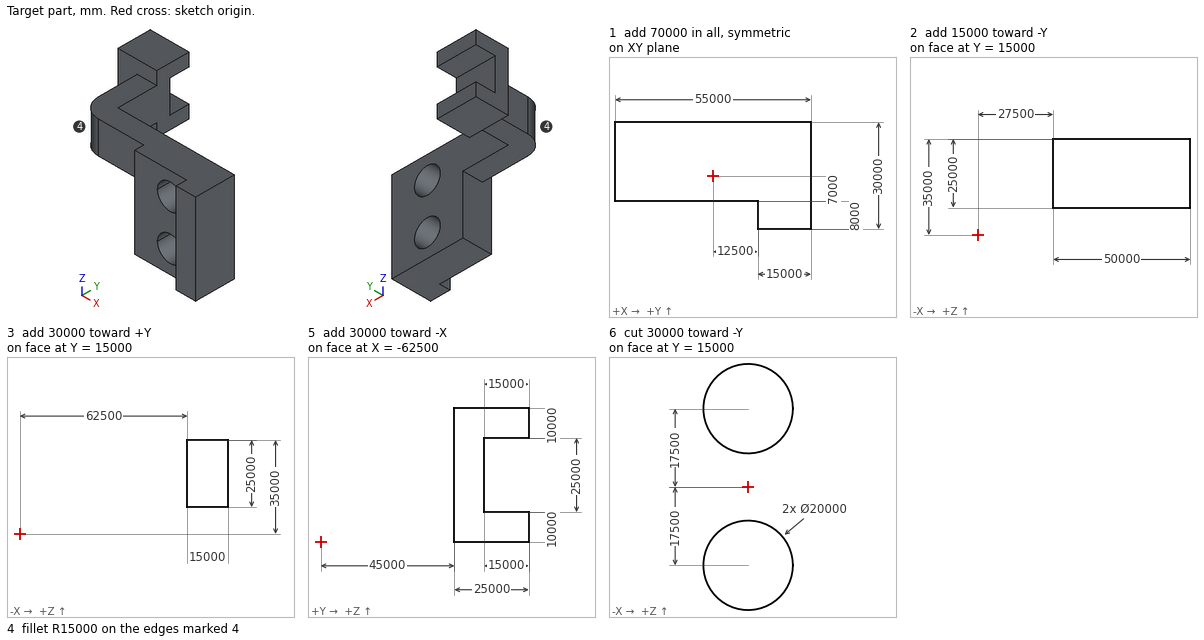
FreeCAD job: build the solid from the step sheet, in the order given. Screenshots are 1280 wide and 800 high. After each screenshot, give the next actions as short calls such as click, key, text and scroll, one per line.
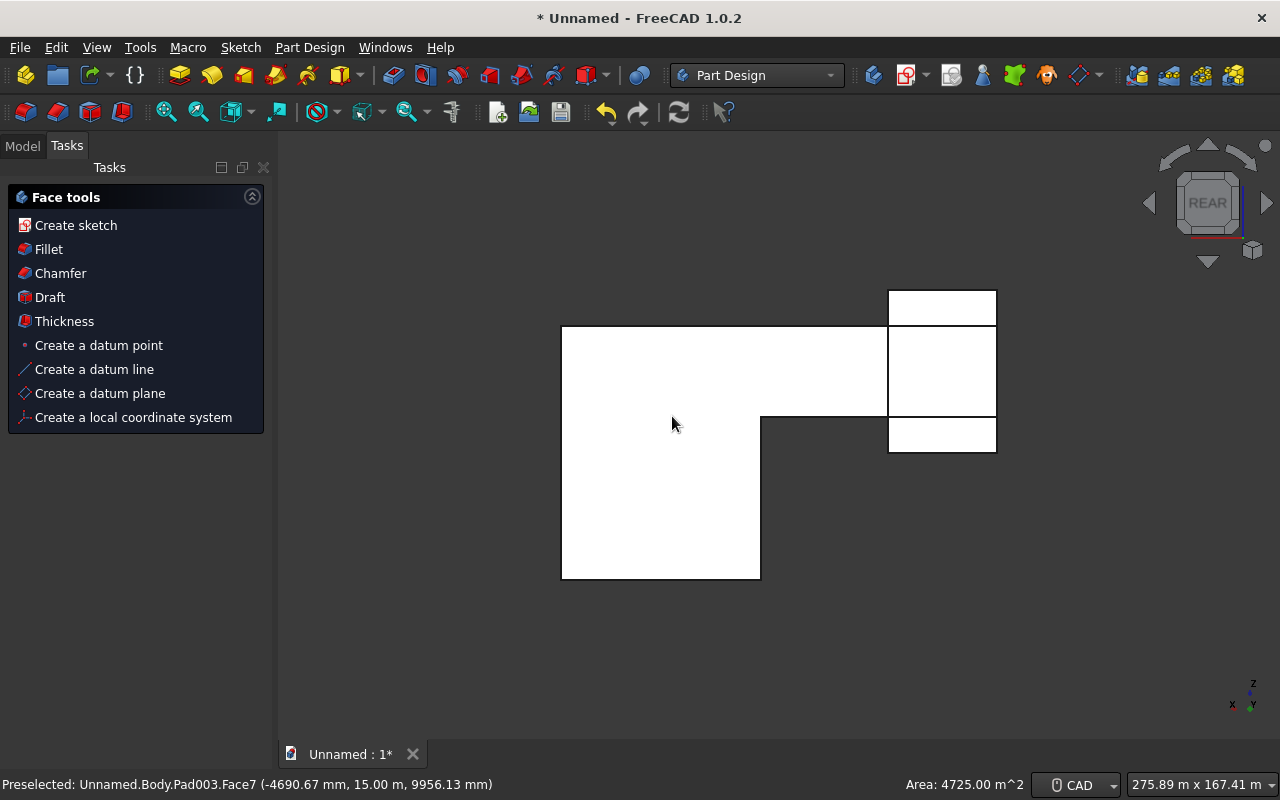
click(906, 76)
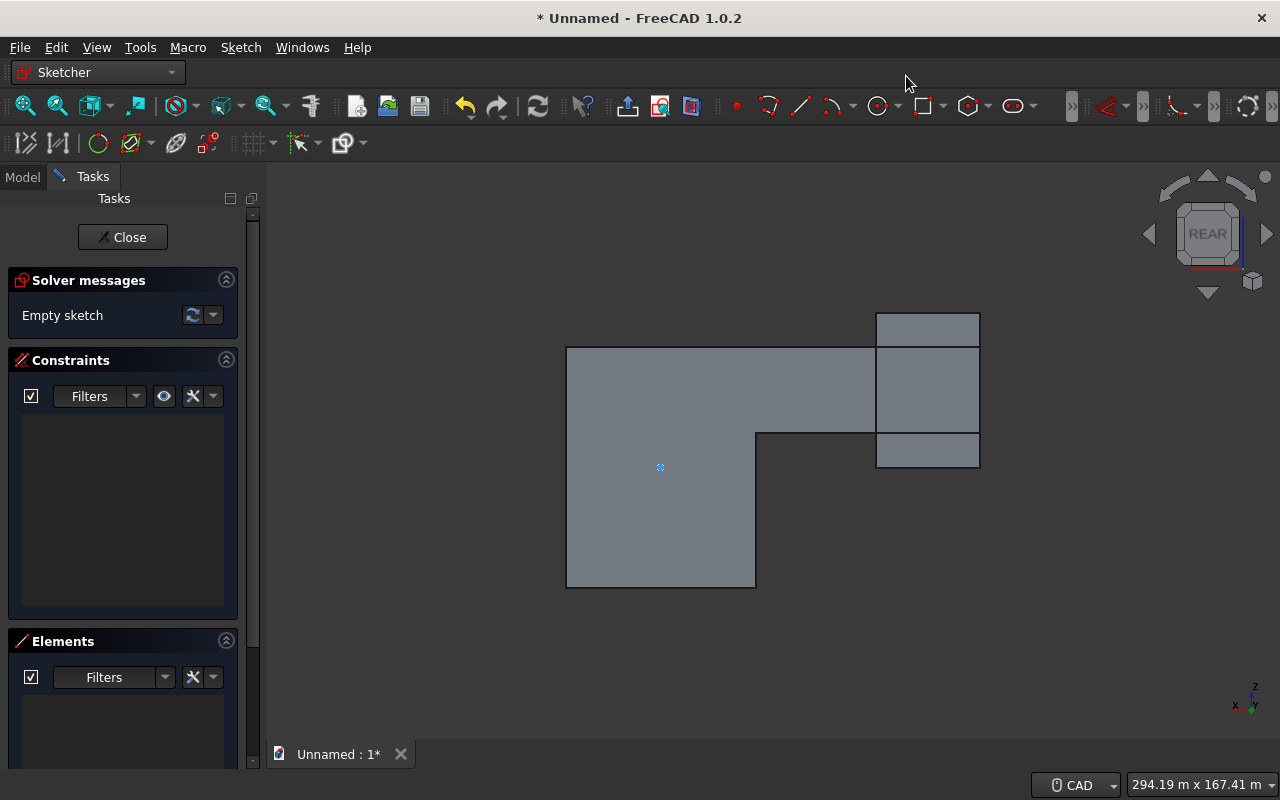
key(q)
key(s)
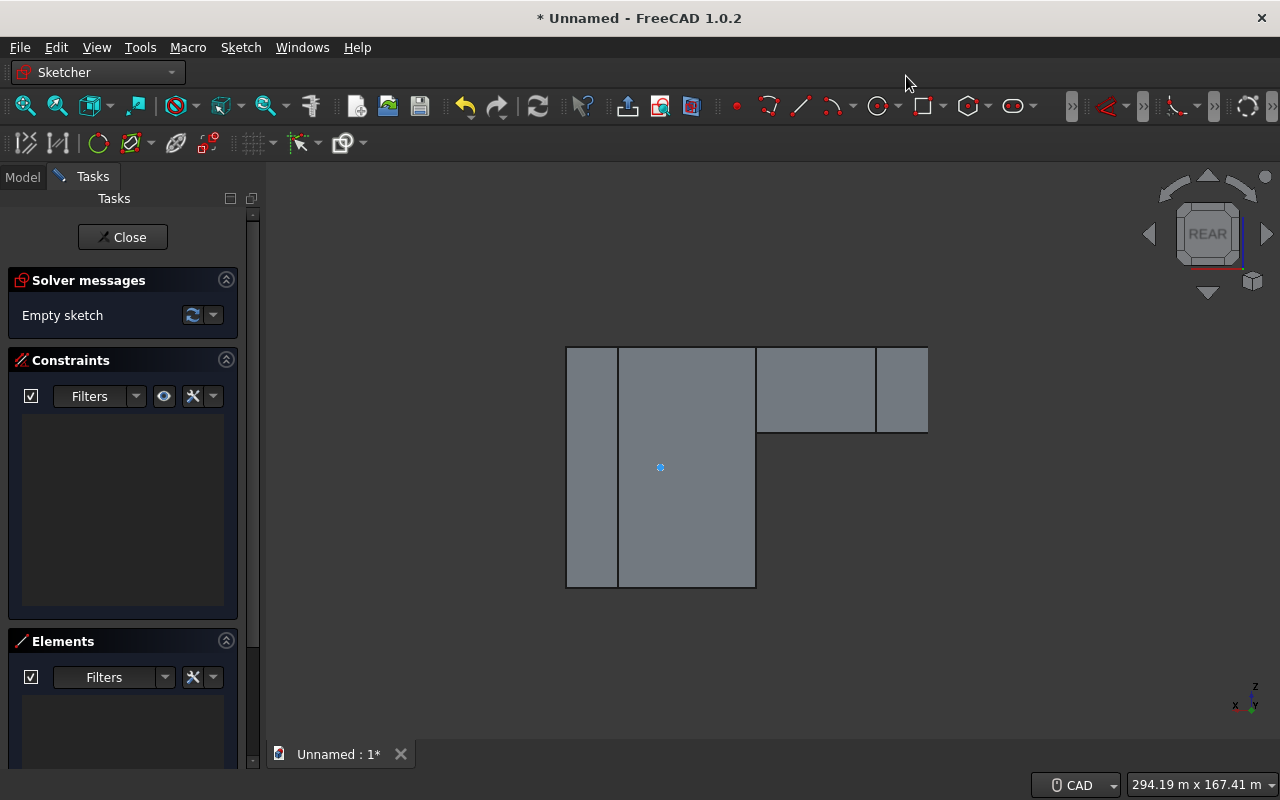
scroll(608, 489, up, 3)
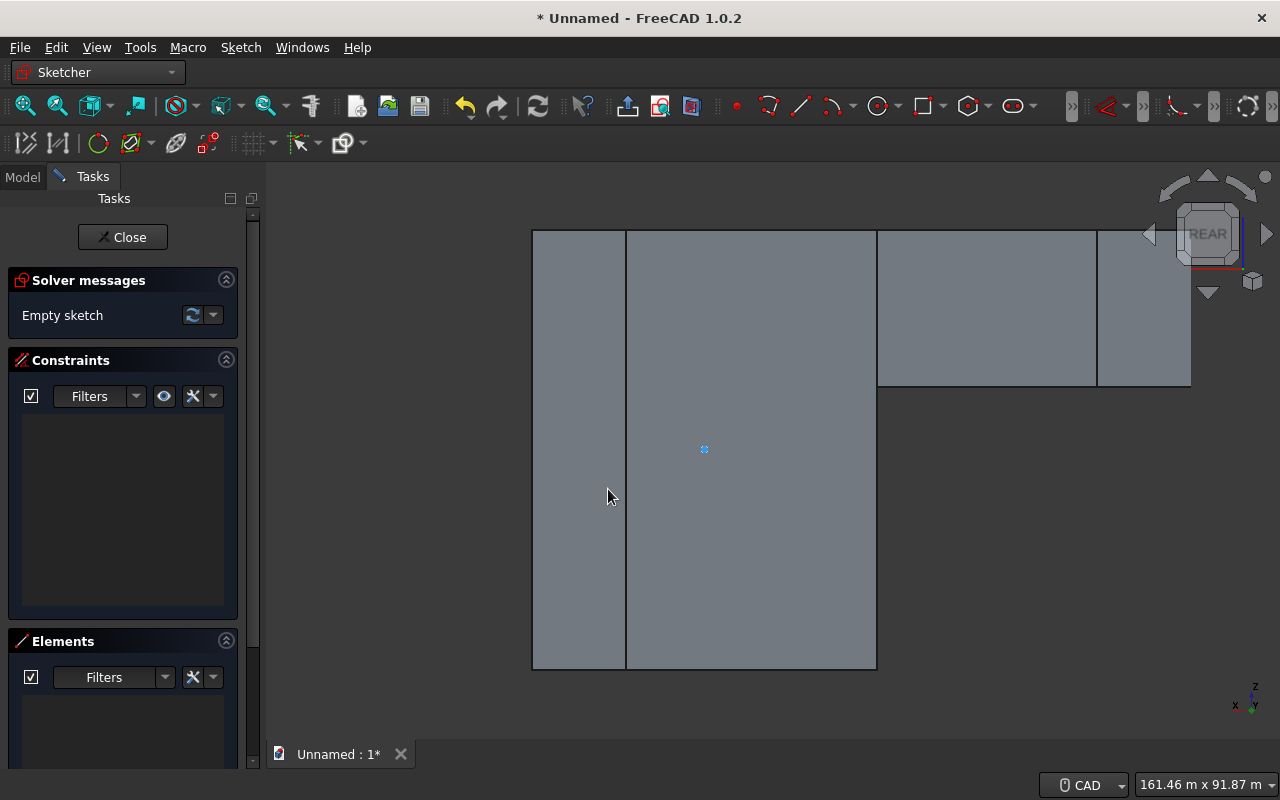
click(878, 106)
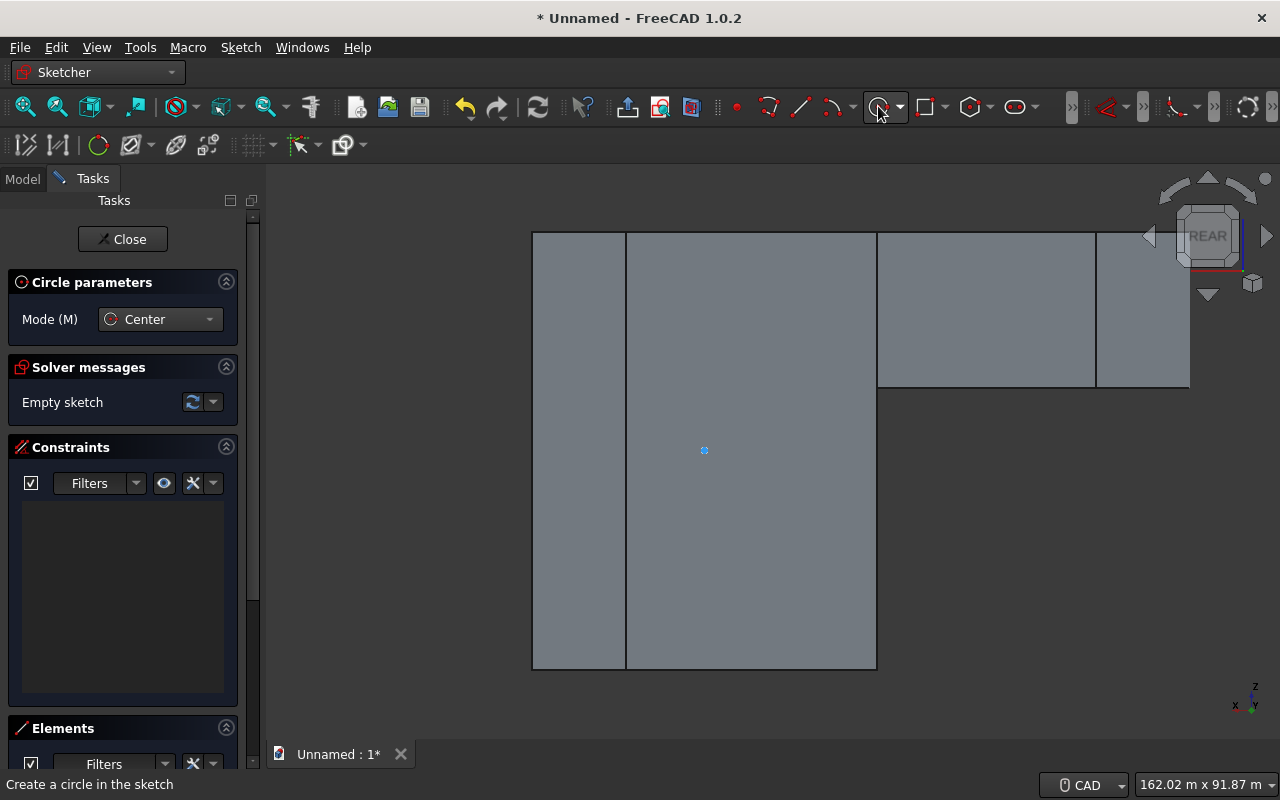
click(705, 560)
click(749, 516)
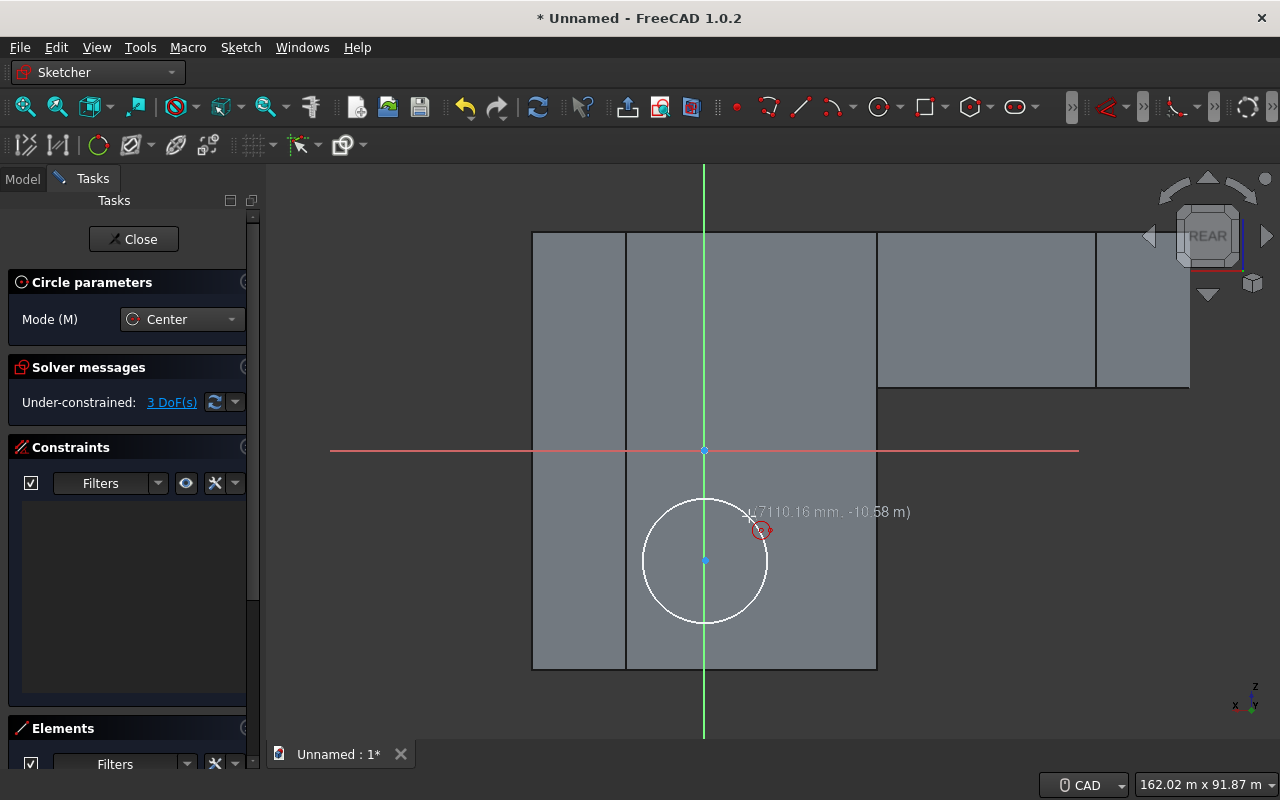
click(705, 341)
click(749, 297)
key(Escape)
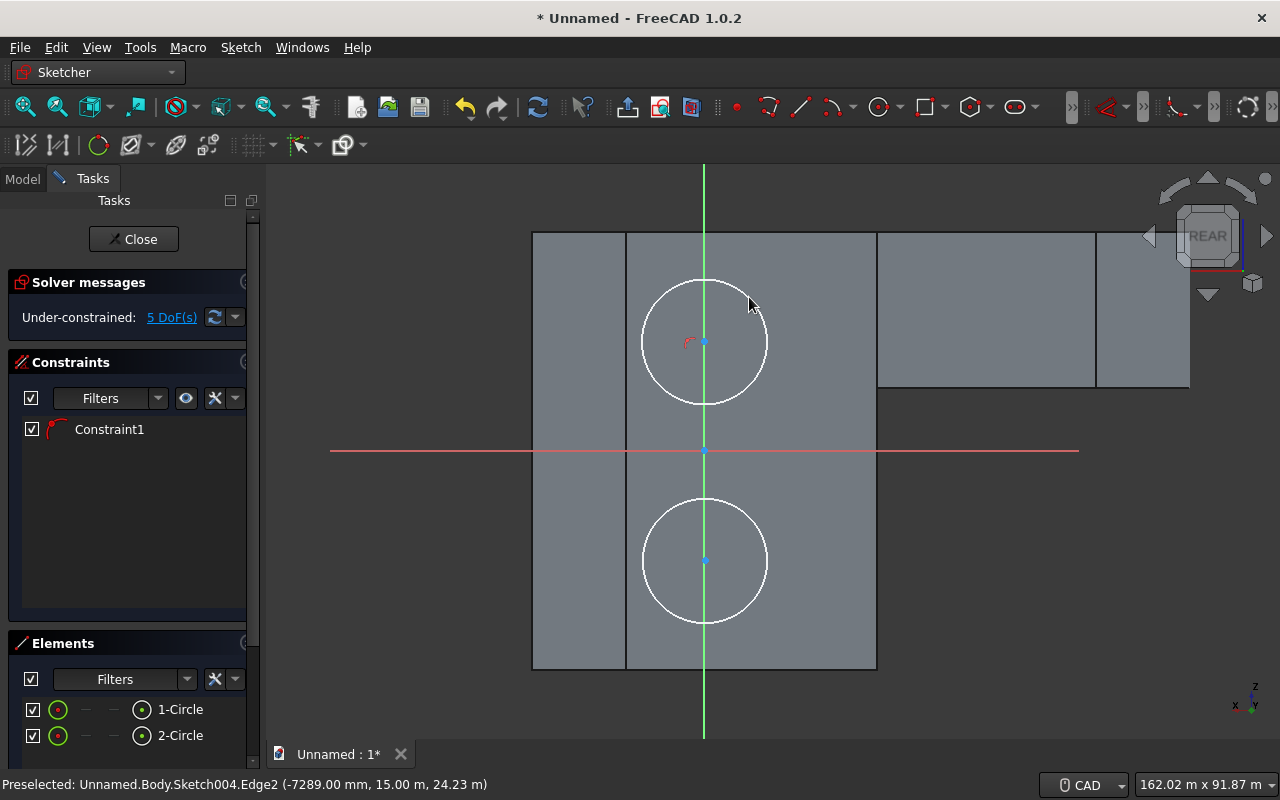
click(749, 517)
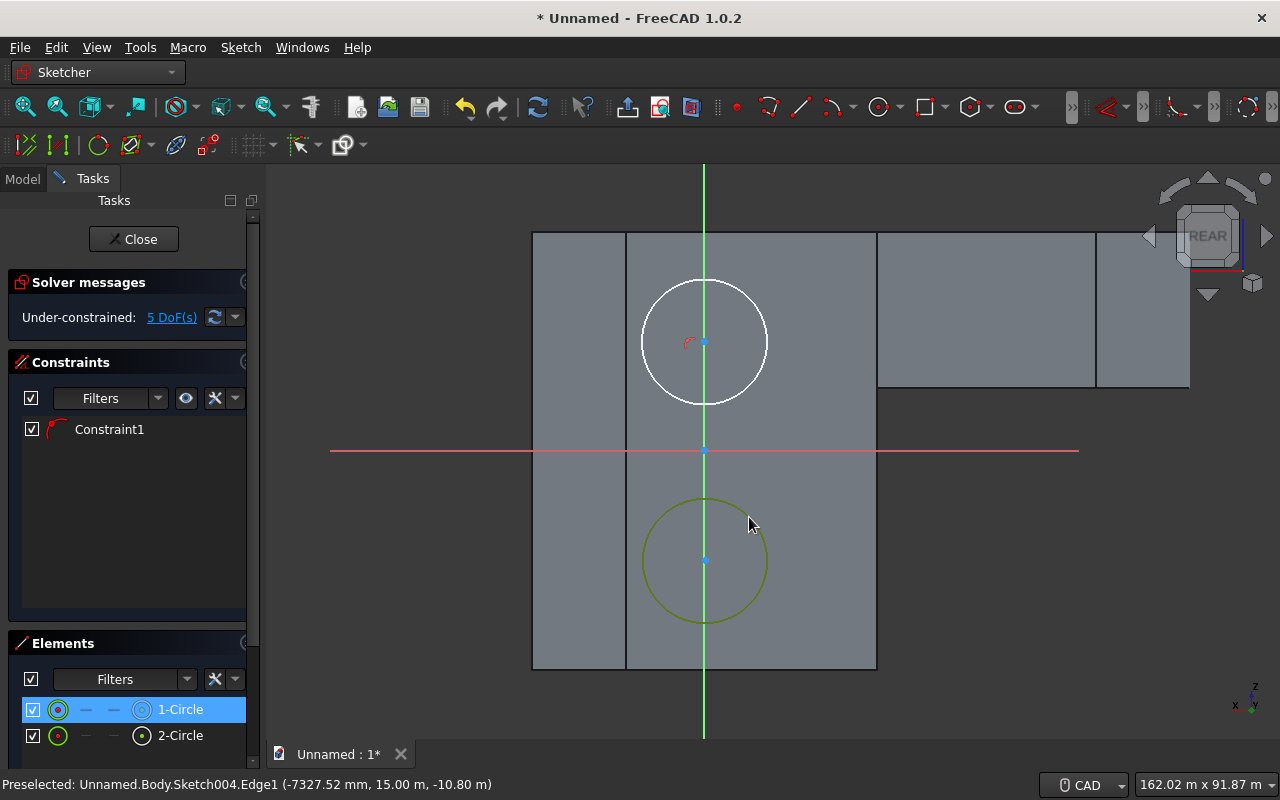
click(749, 298)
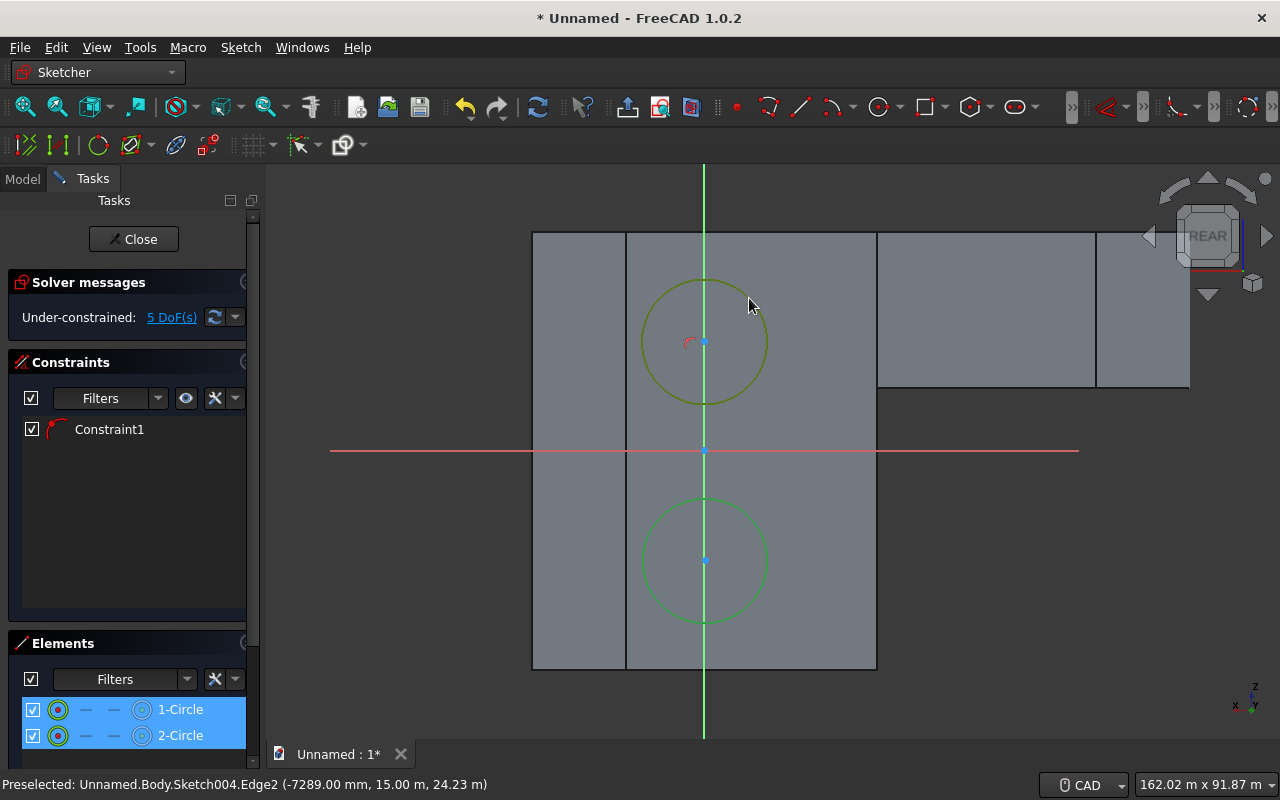
key(e)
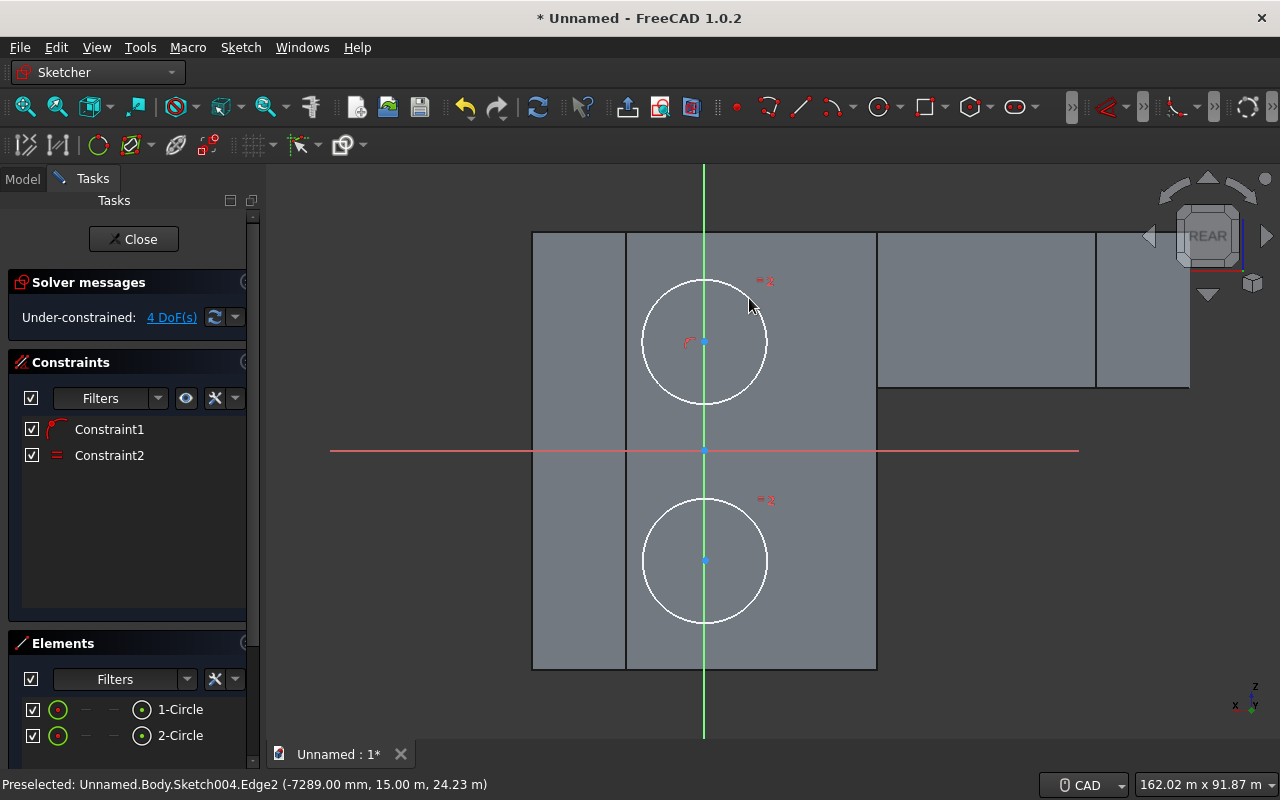
click(705, 561)